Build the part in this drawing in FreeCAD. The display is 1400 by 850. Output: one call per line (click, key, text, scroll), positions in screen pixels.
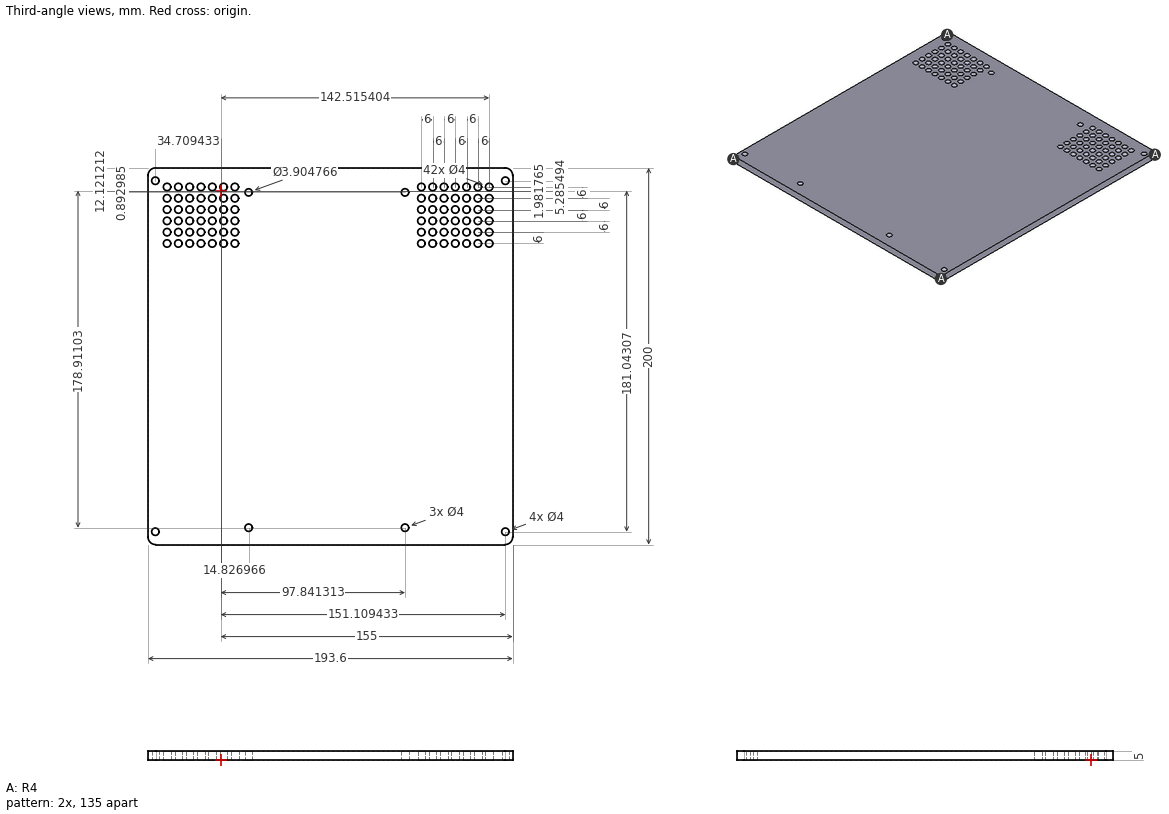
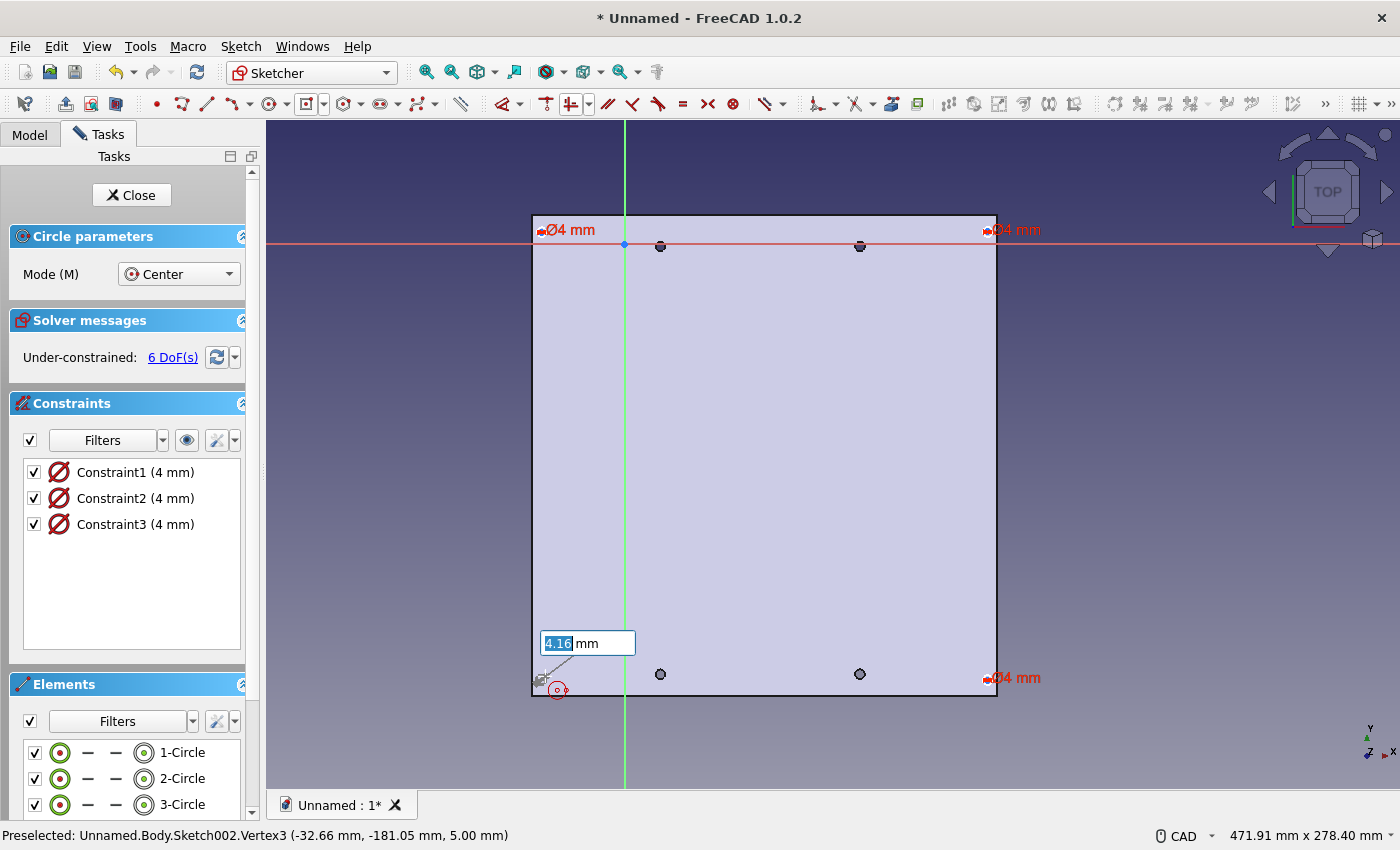
text(4)
key(Return)
key(Escape)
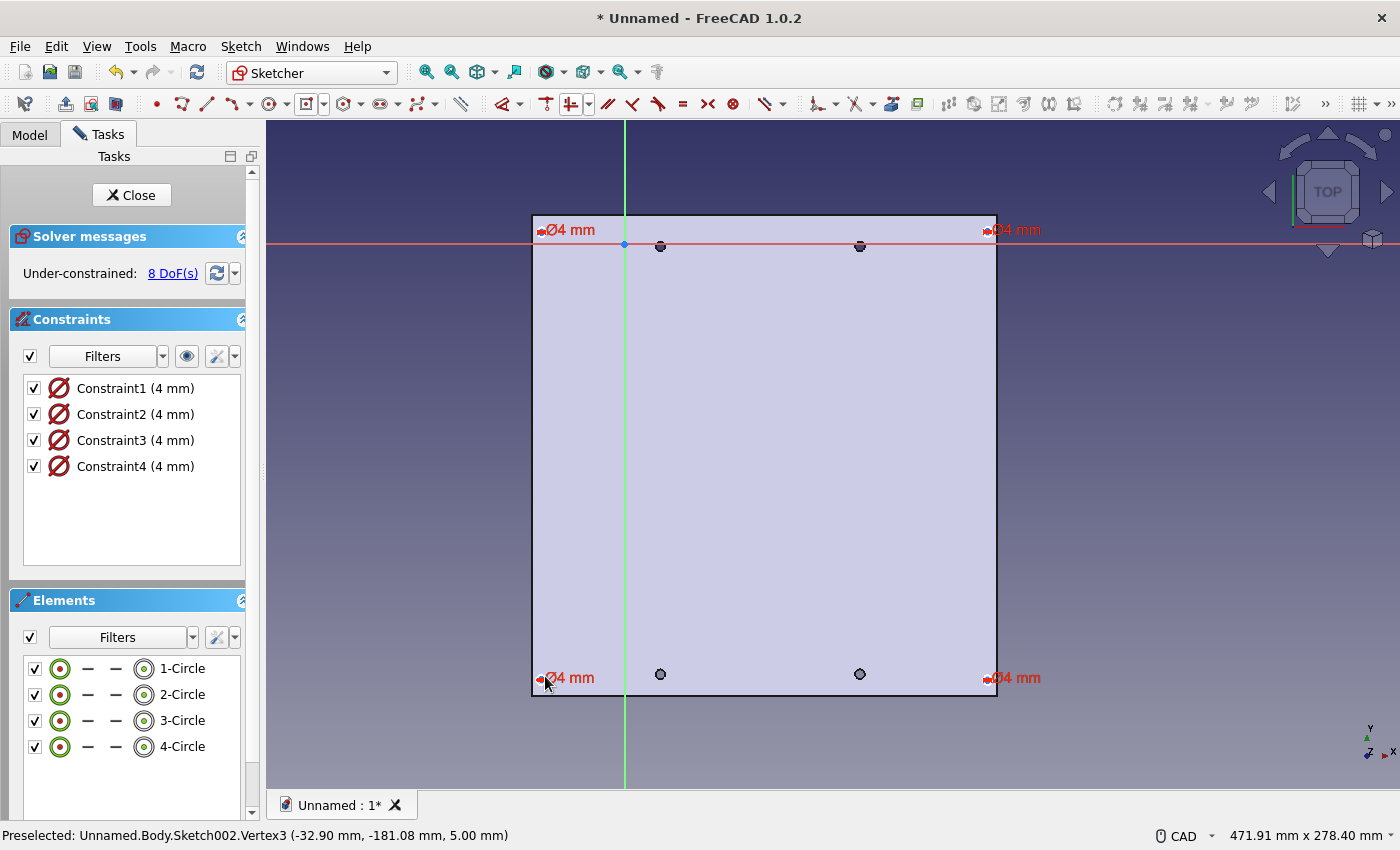
click(502, 104)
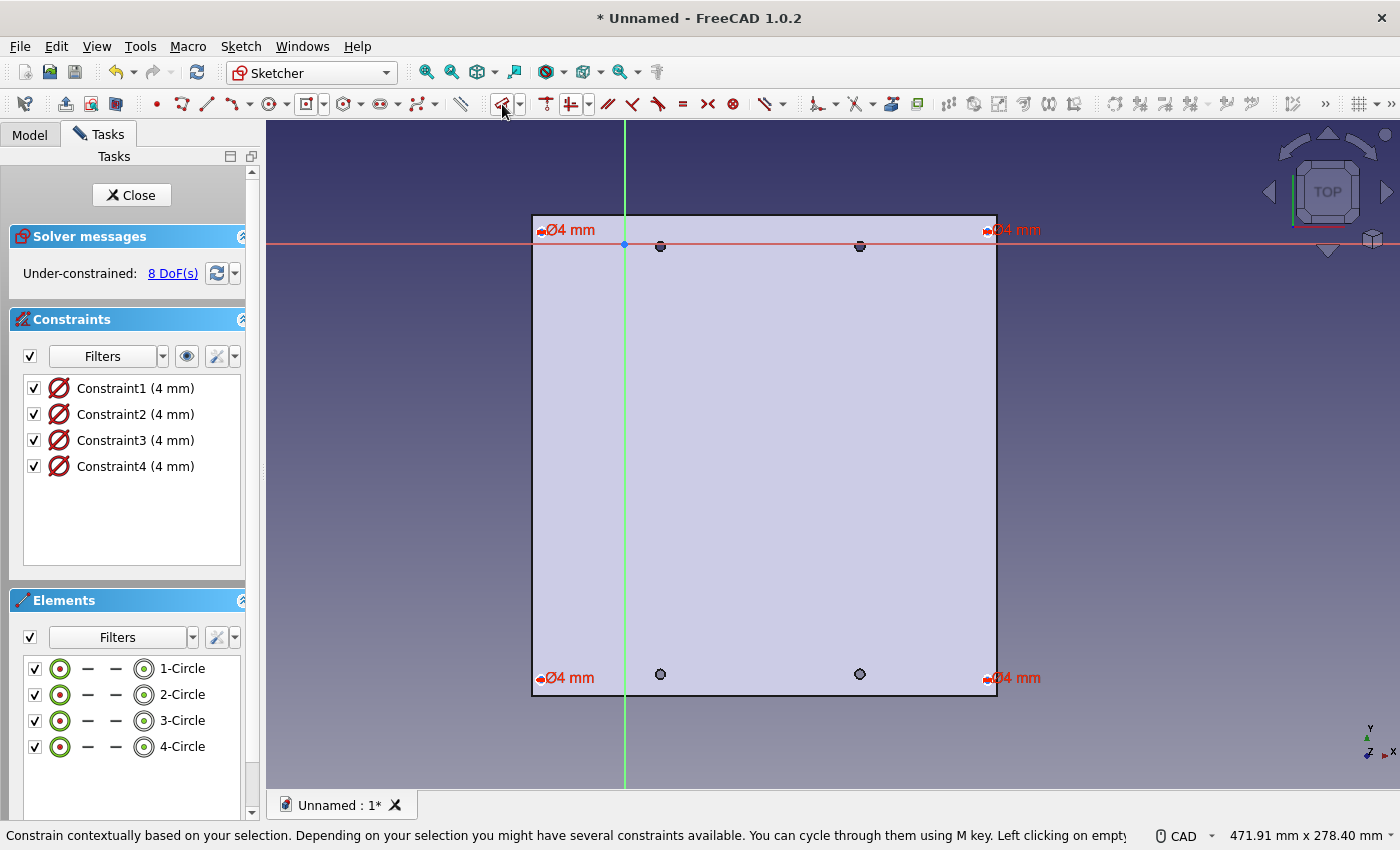
scroll(988, 232, up, 6)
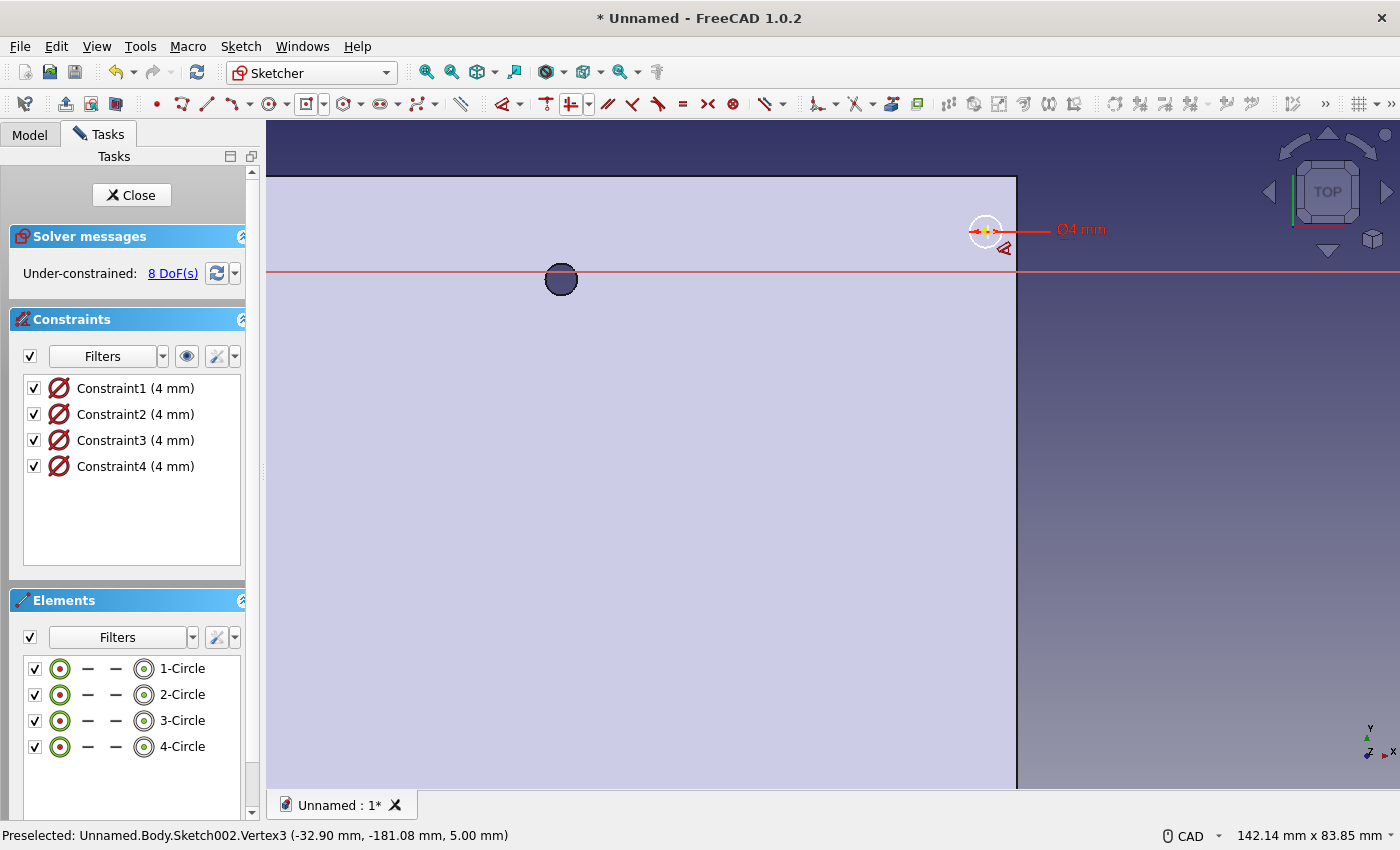
click(986, 232)
click(1020, 252)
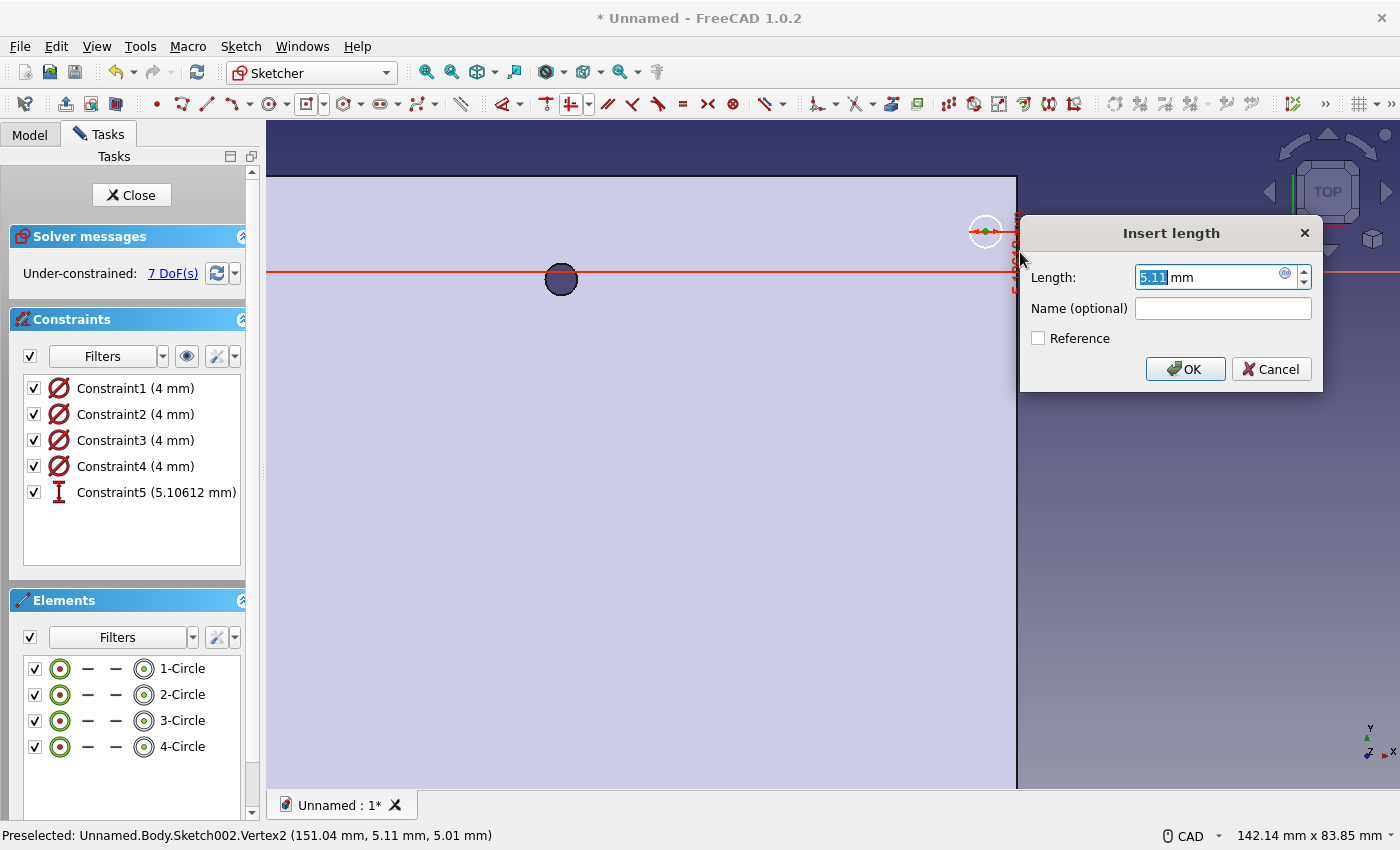
text(5.285494)
key(Return)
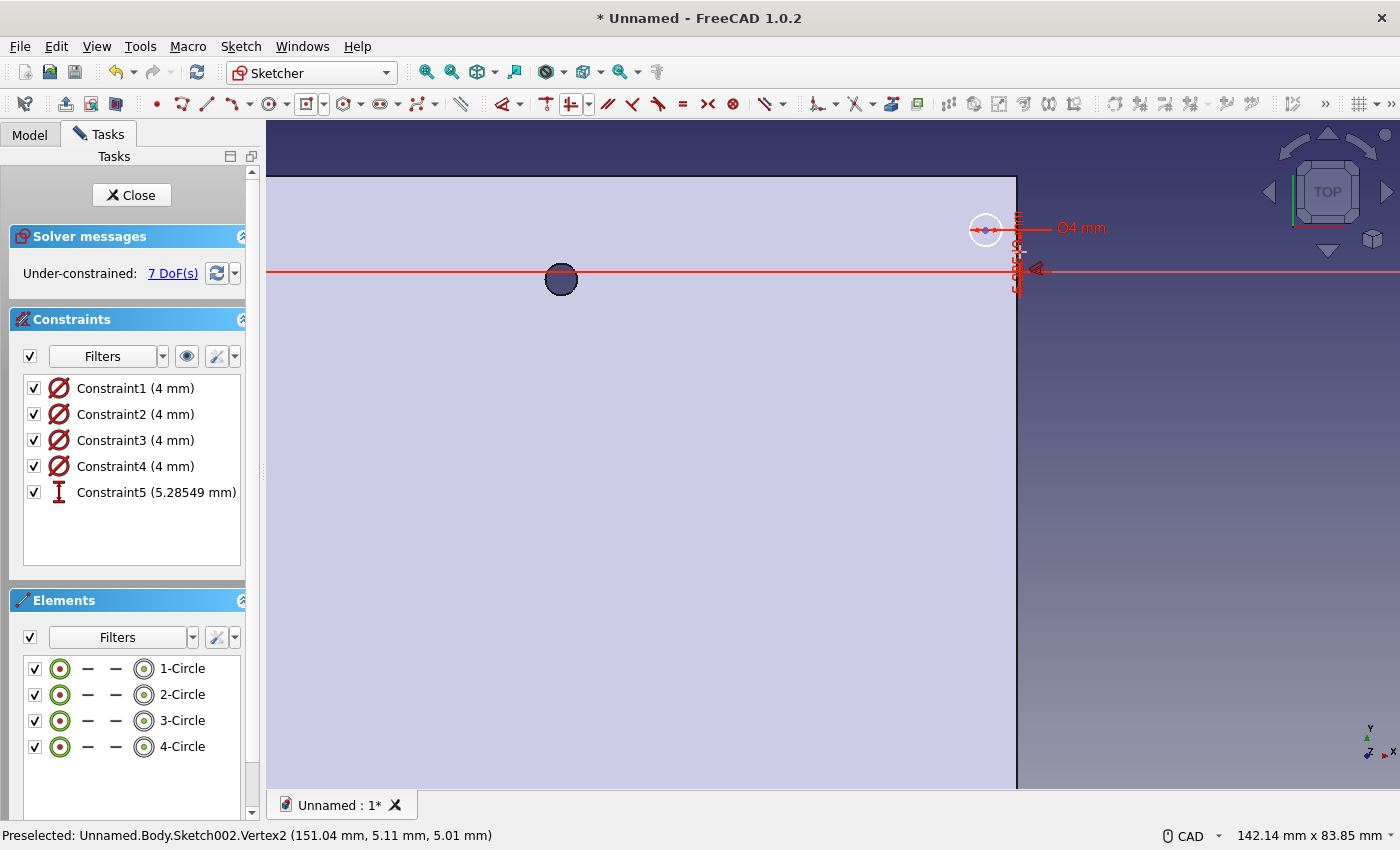
scroll(988, 231, down, 6)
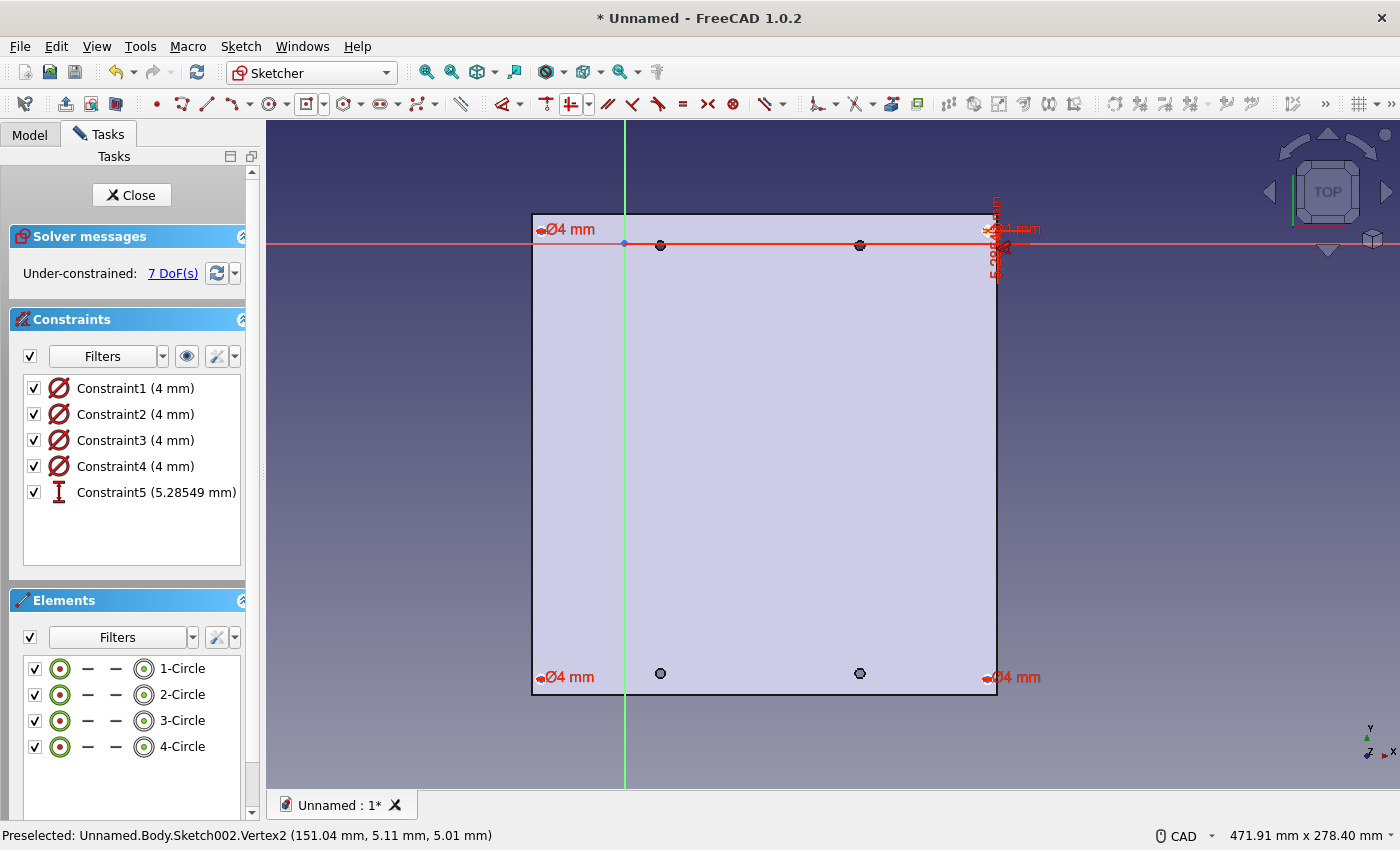
scroll(542, 231, up, 6)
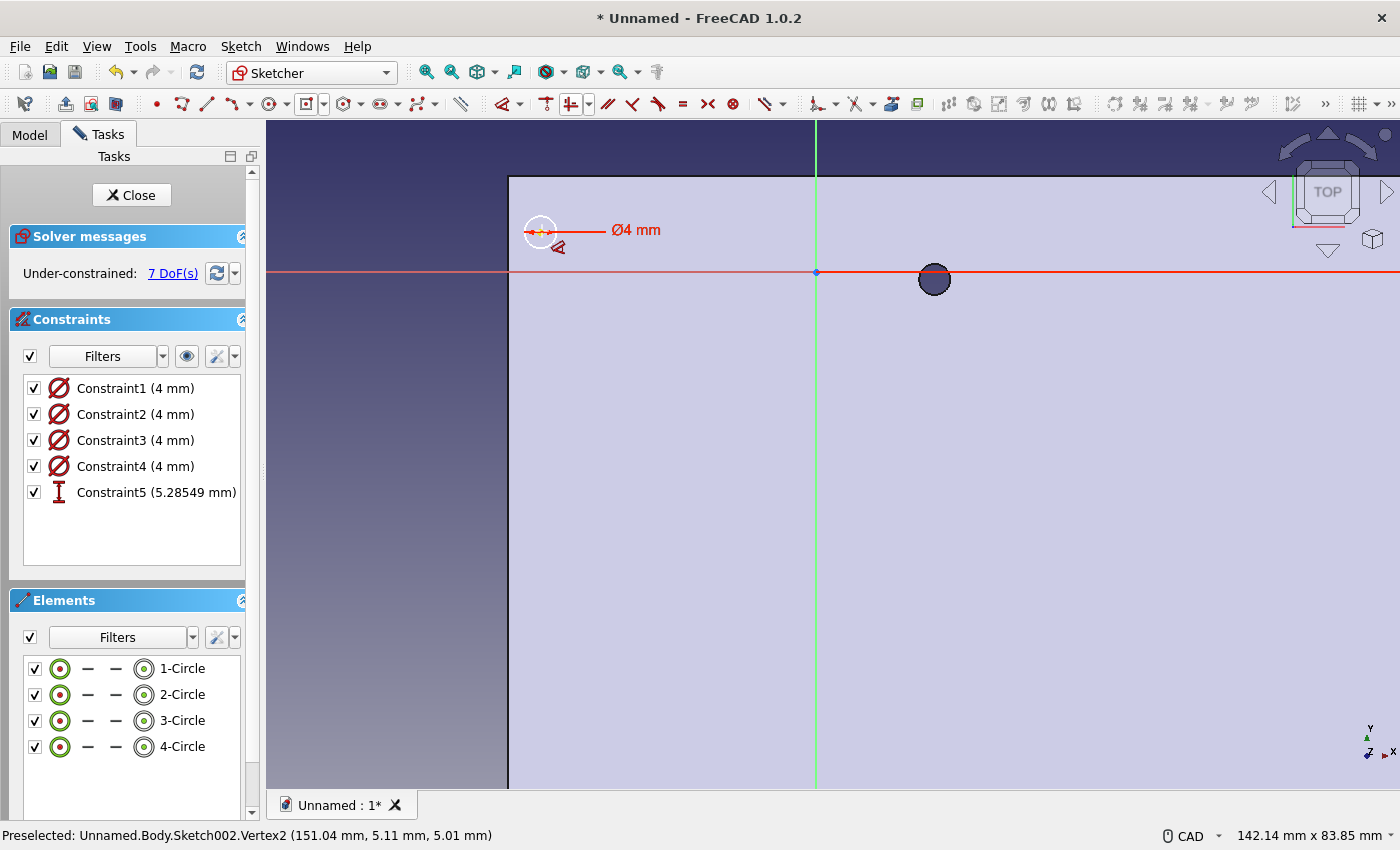
click(541, 232)
click(507, 252)